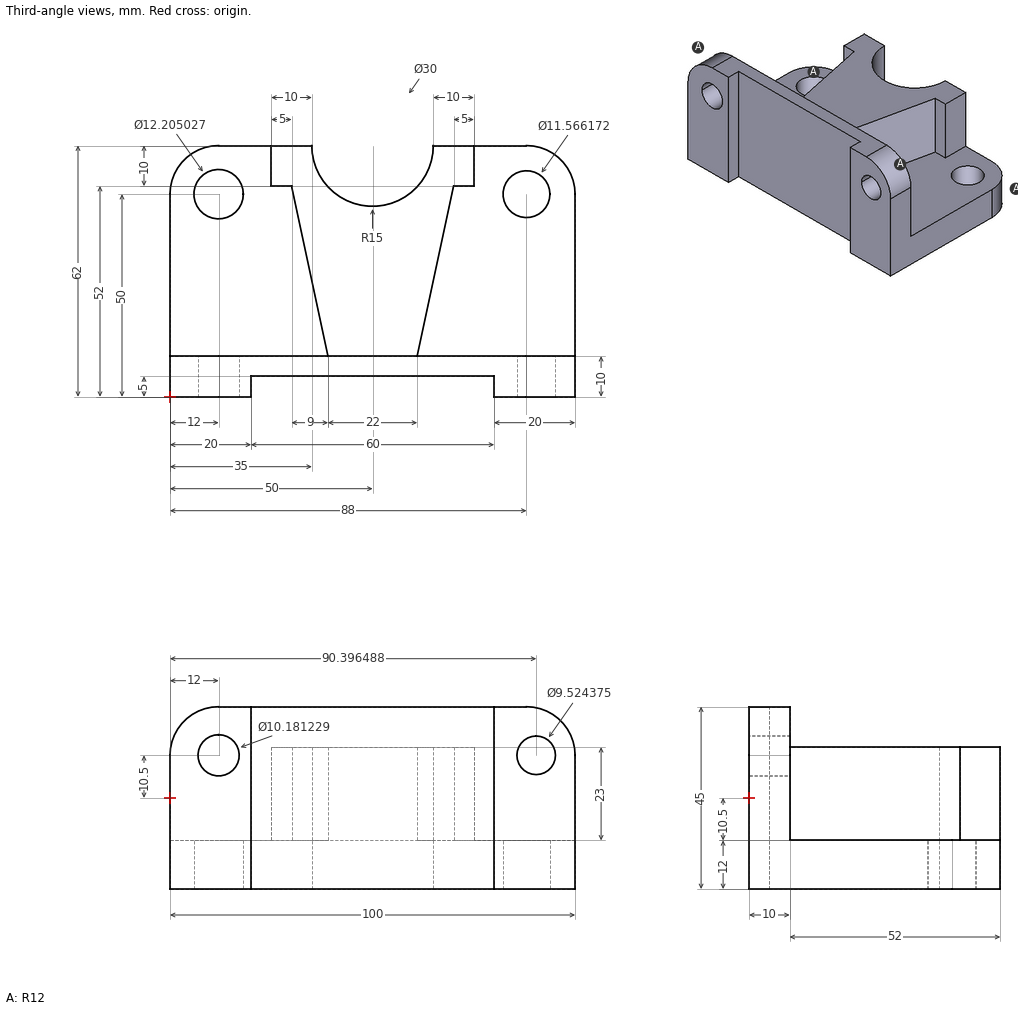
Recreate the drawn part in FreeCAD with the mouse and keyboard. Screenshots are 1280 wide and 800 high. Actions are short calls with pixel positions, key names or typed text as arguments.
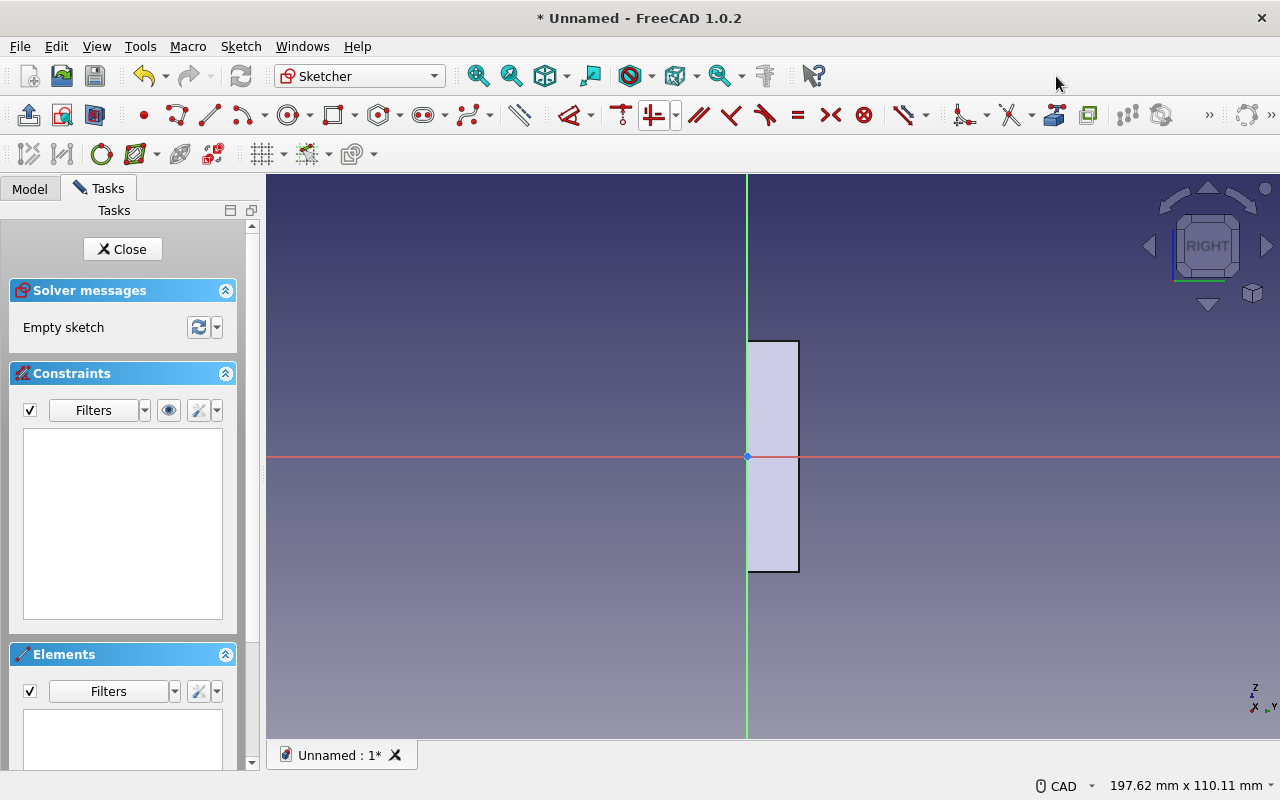
scroll(1115, 584, up, 3)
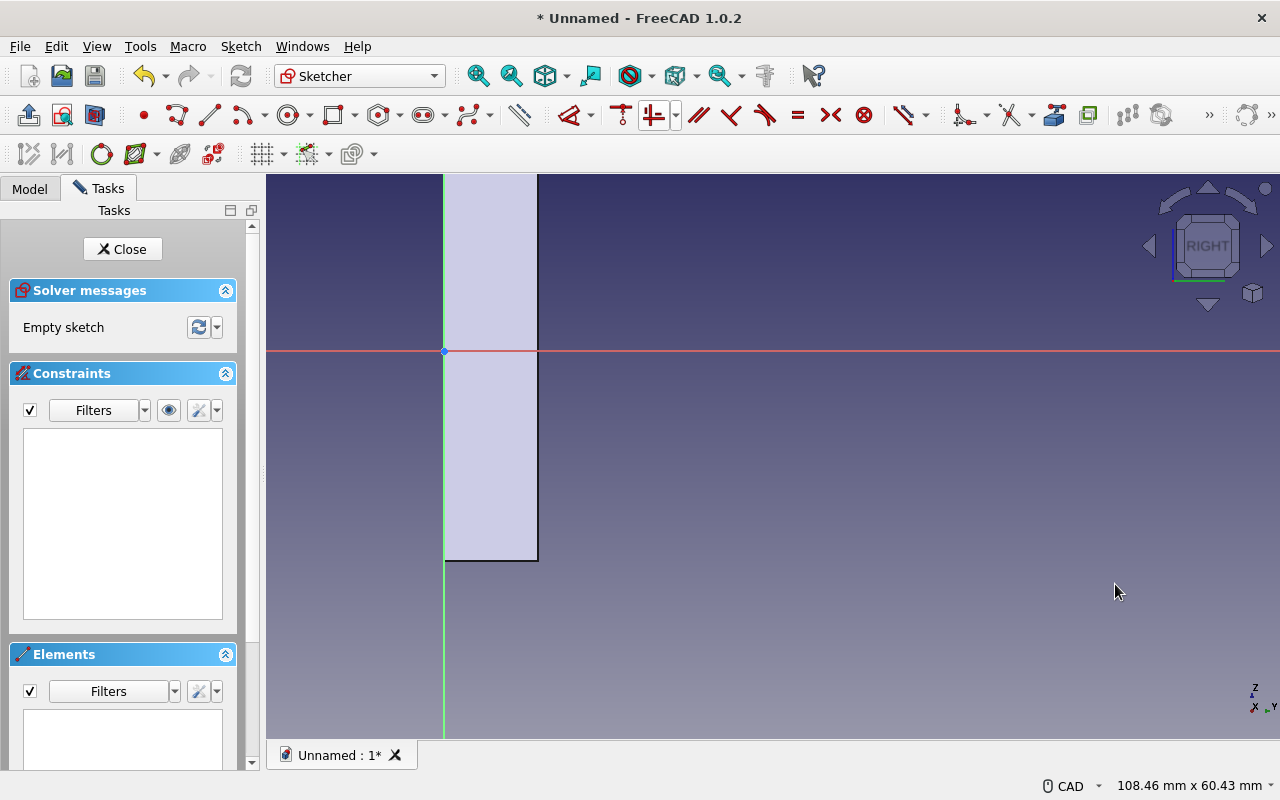
key(g)
key(r)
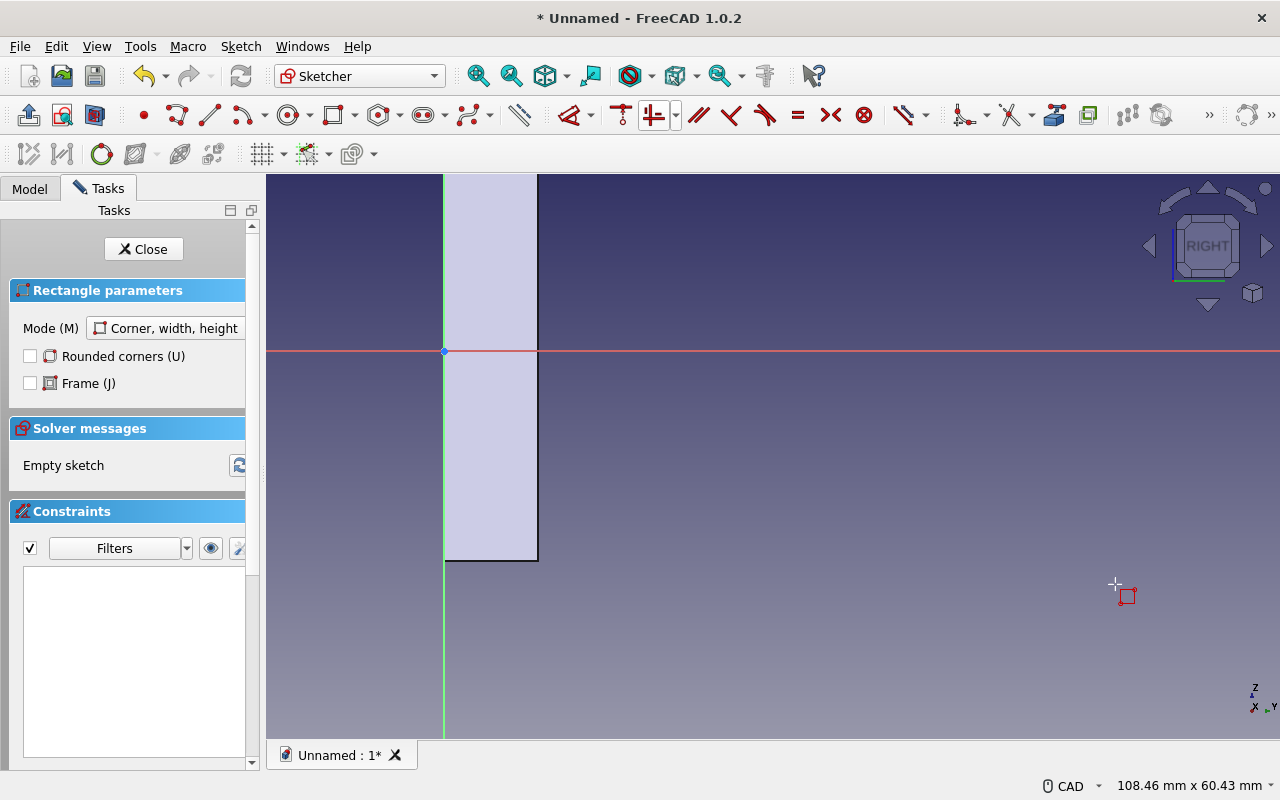
click(538, 449)
click(1024, 561)
key(Escape)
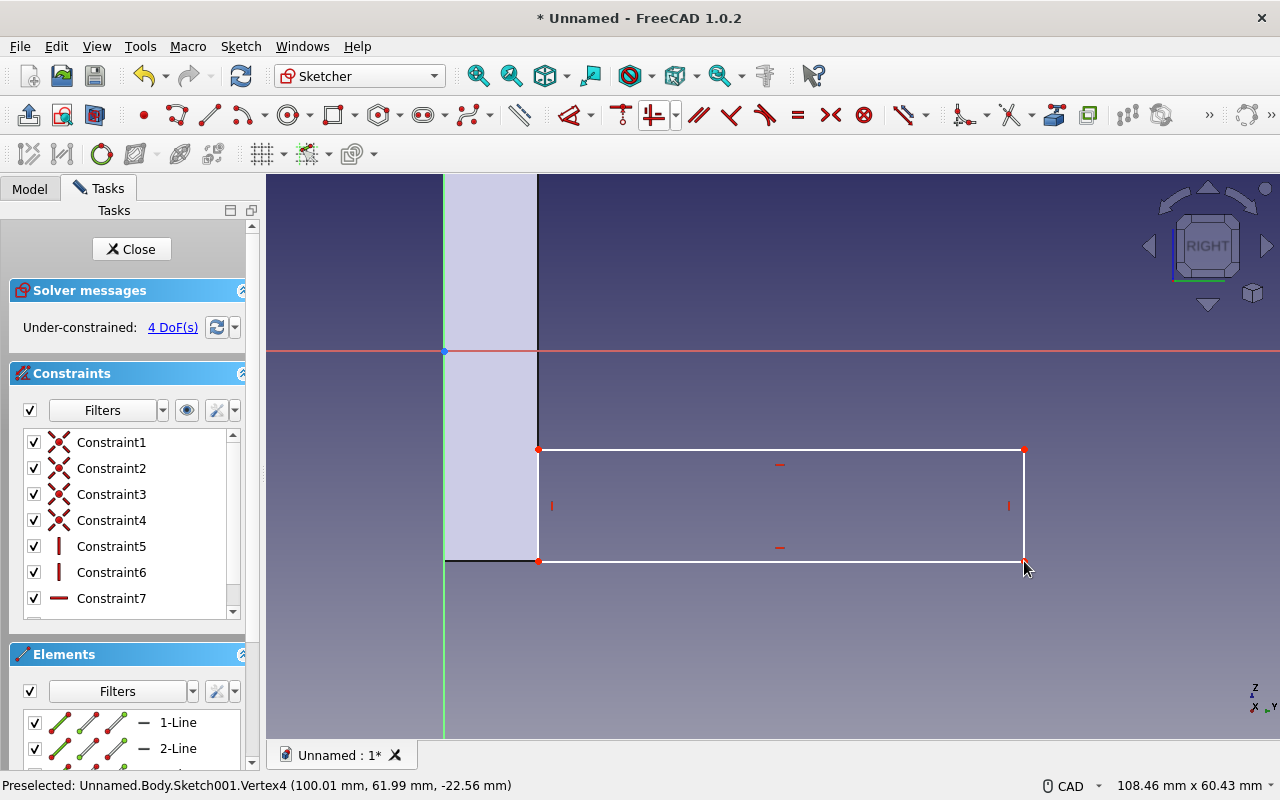
click(538, 484)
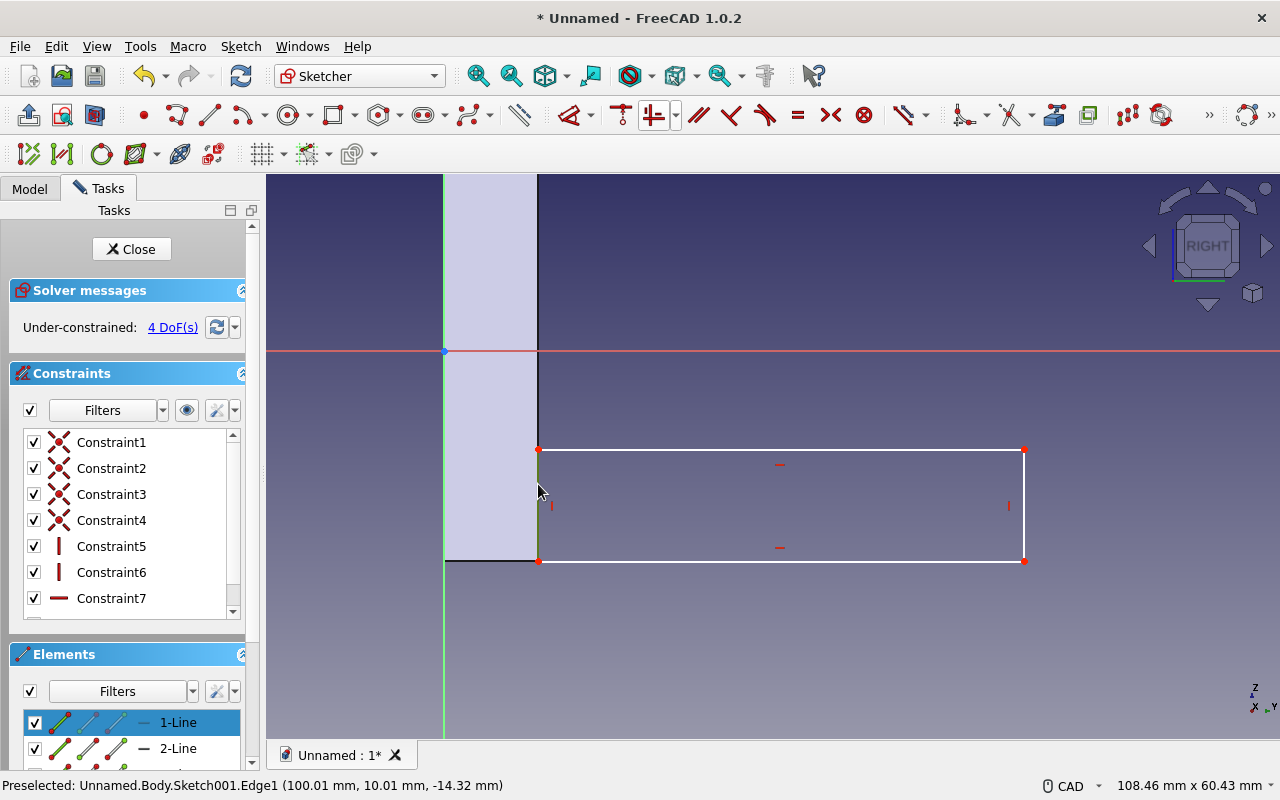
key(i)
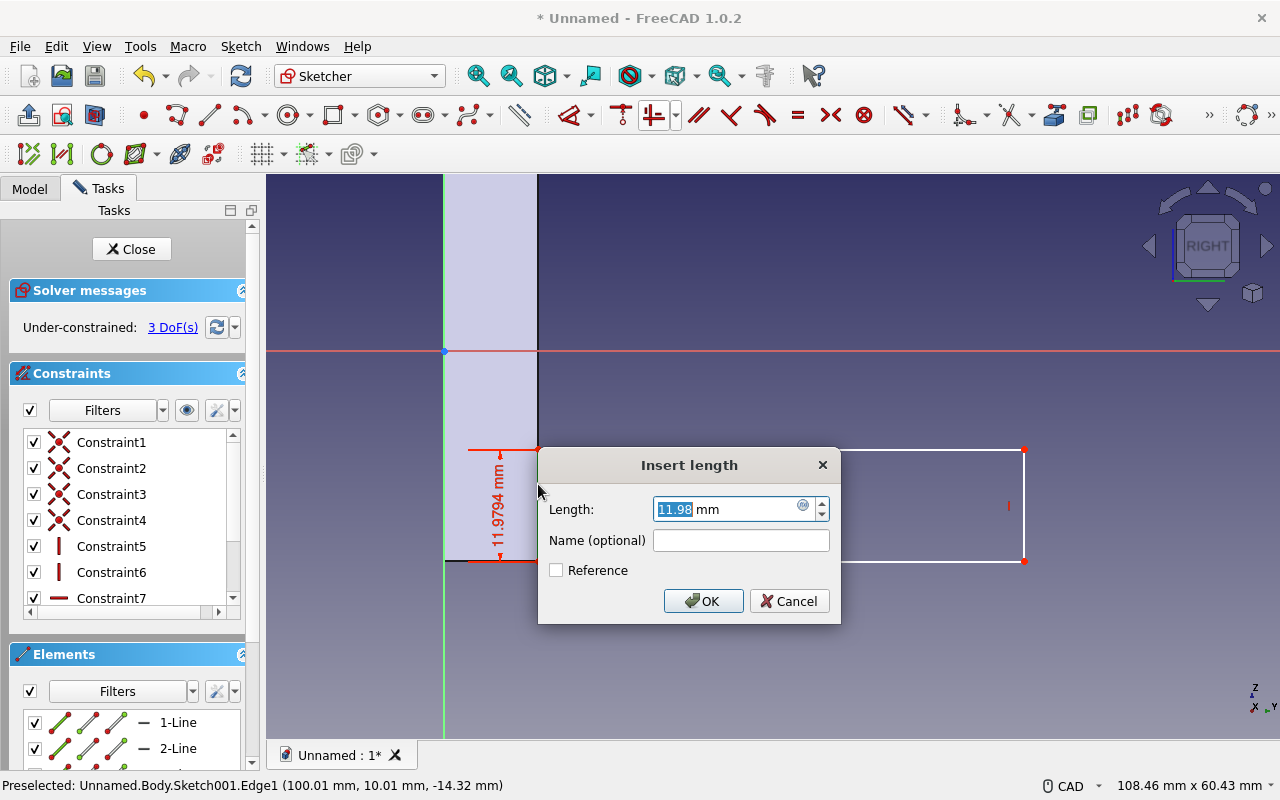
text(12)
key(Return)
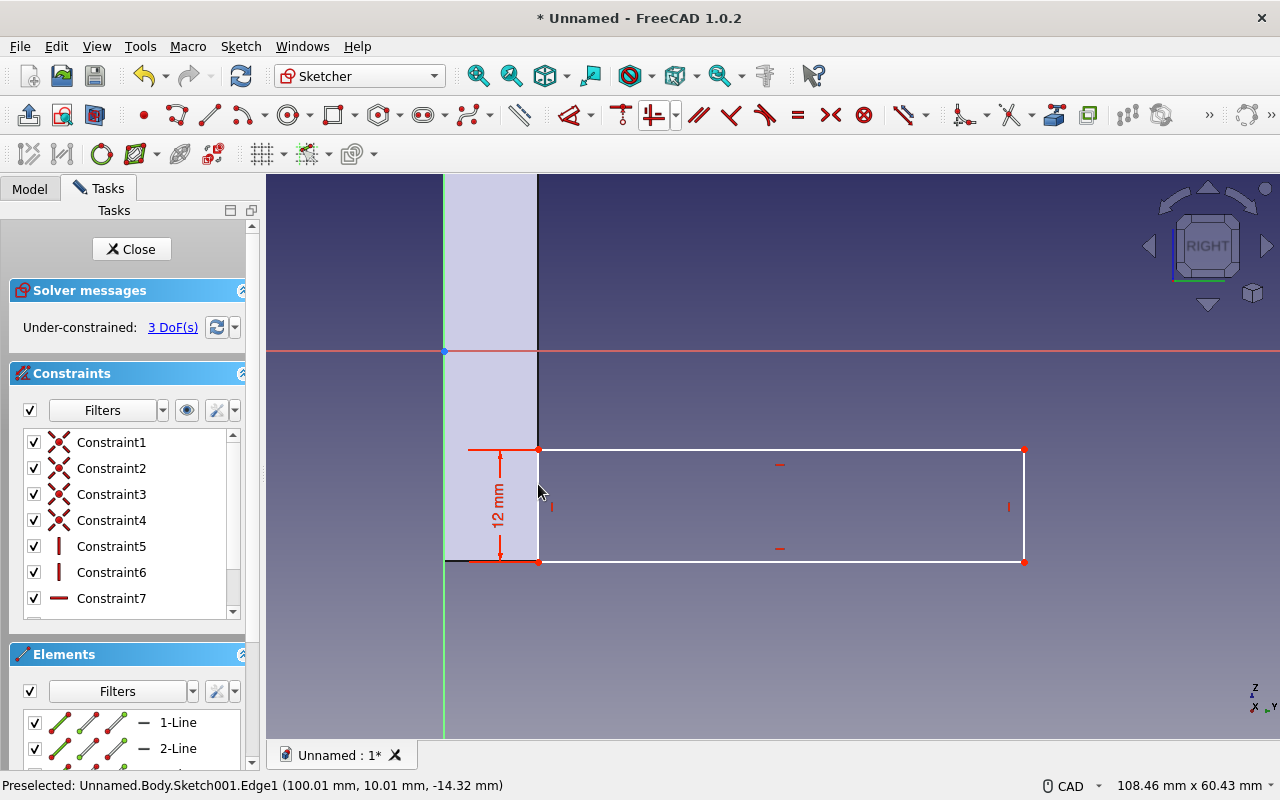
click(684, 562)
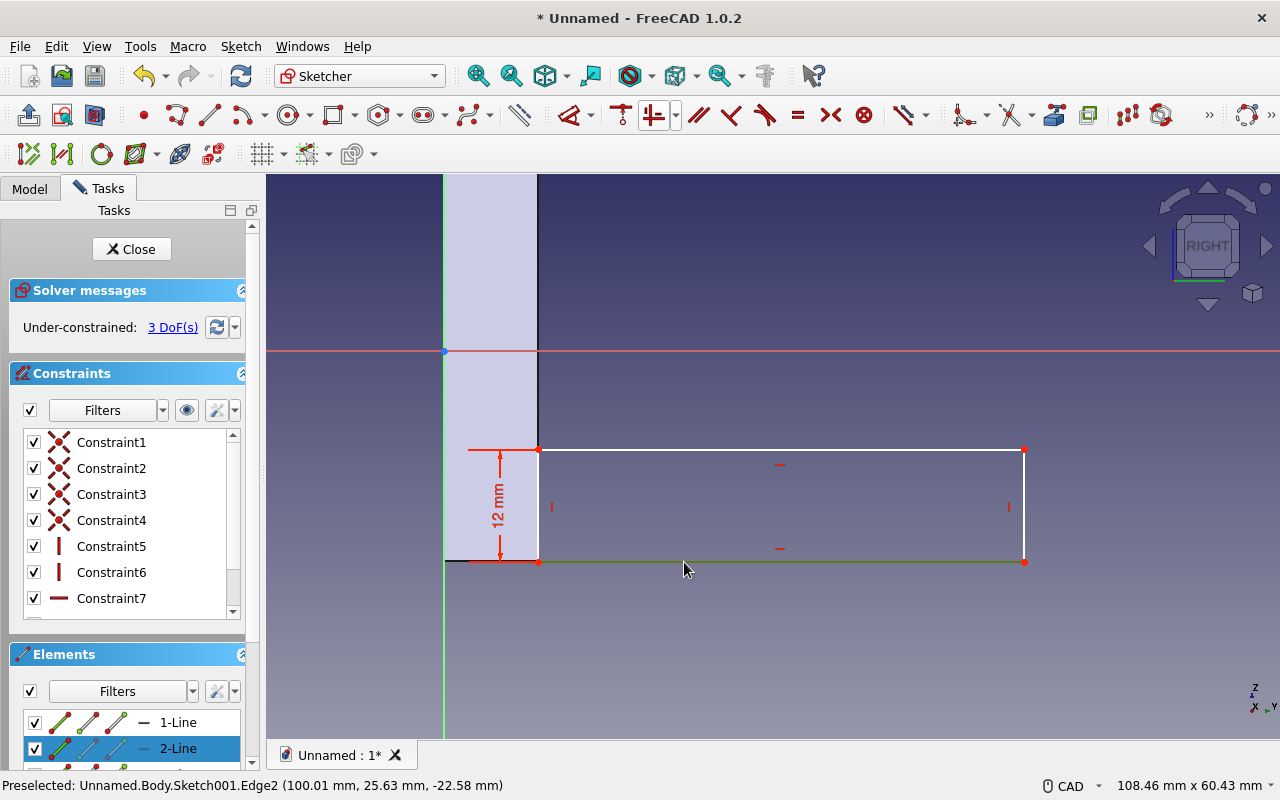
key(l)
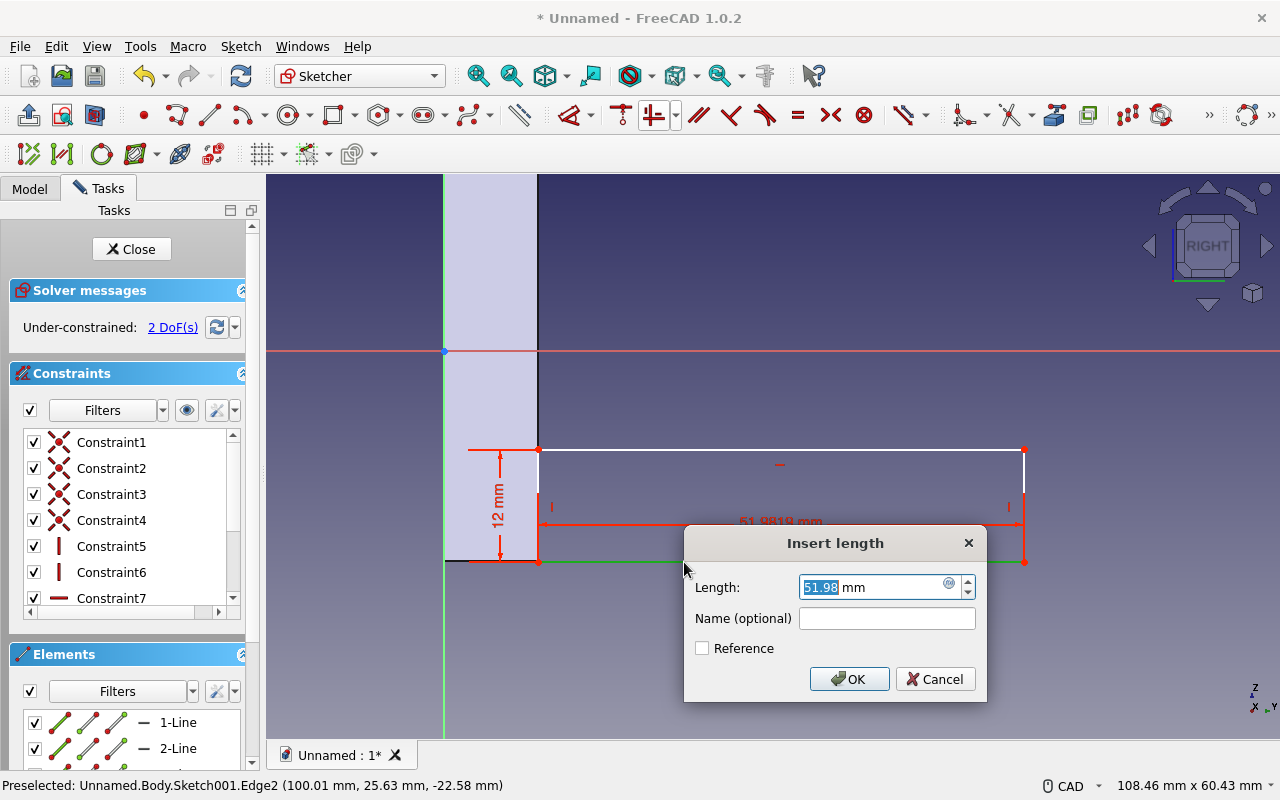
text(52)
key(Return)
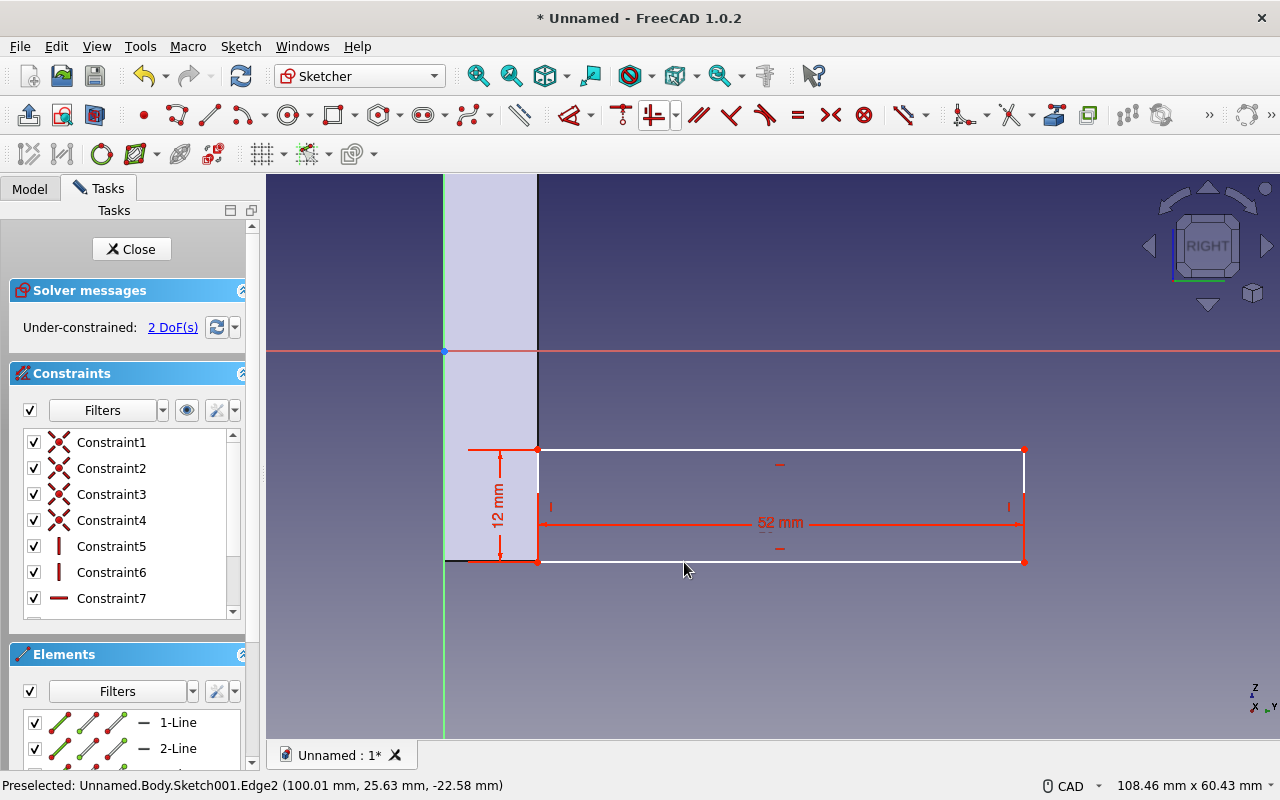
click(538, 450)